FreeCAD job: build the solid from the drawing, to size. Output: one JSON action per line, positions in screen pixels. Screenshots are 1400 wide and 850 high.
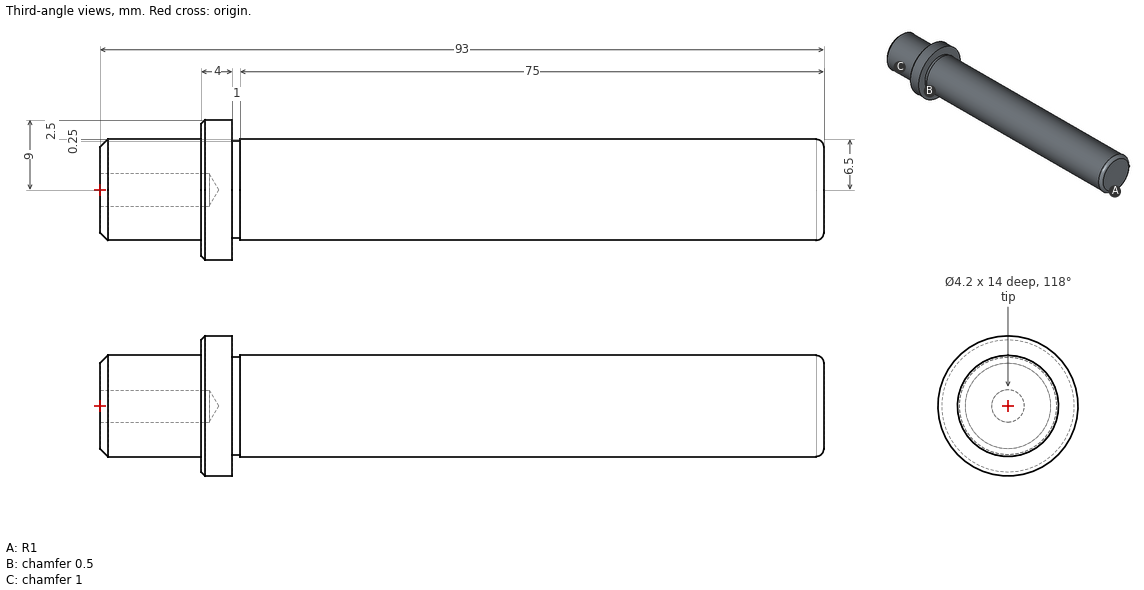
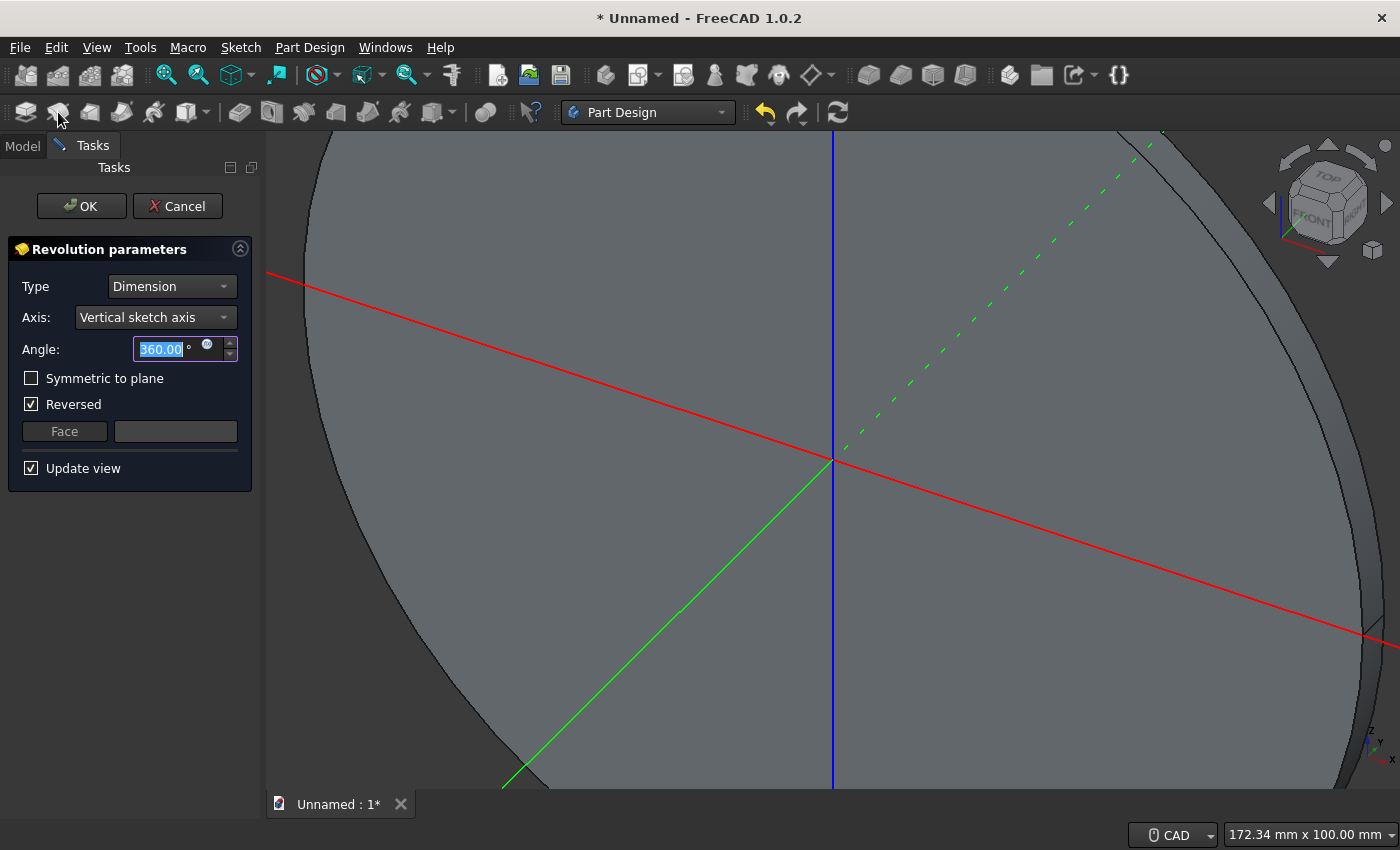
{"action": "left_click", "coordinate": [156, 318]}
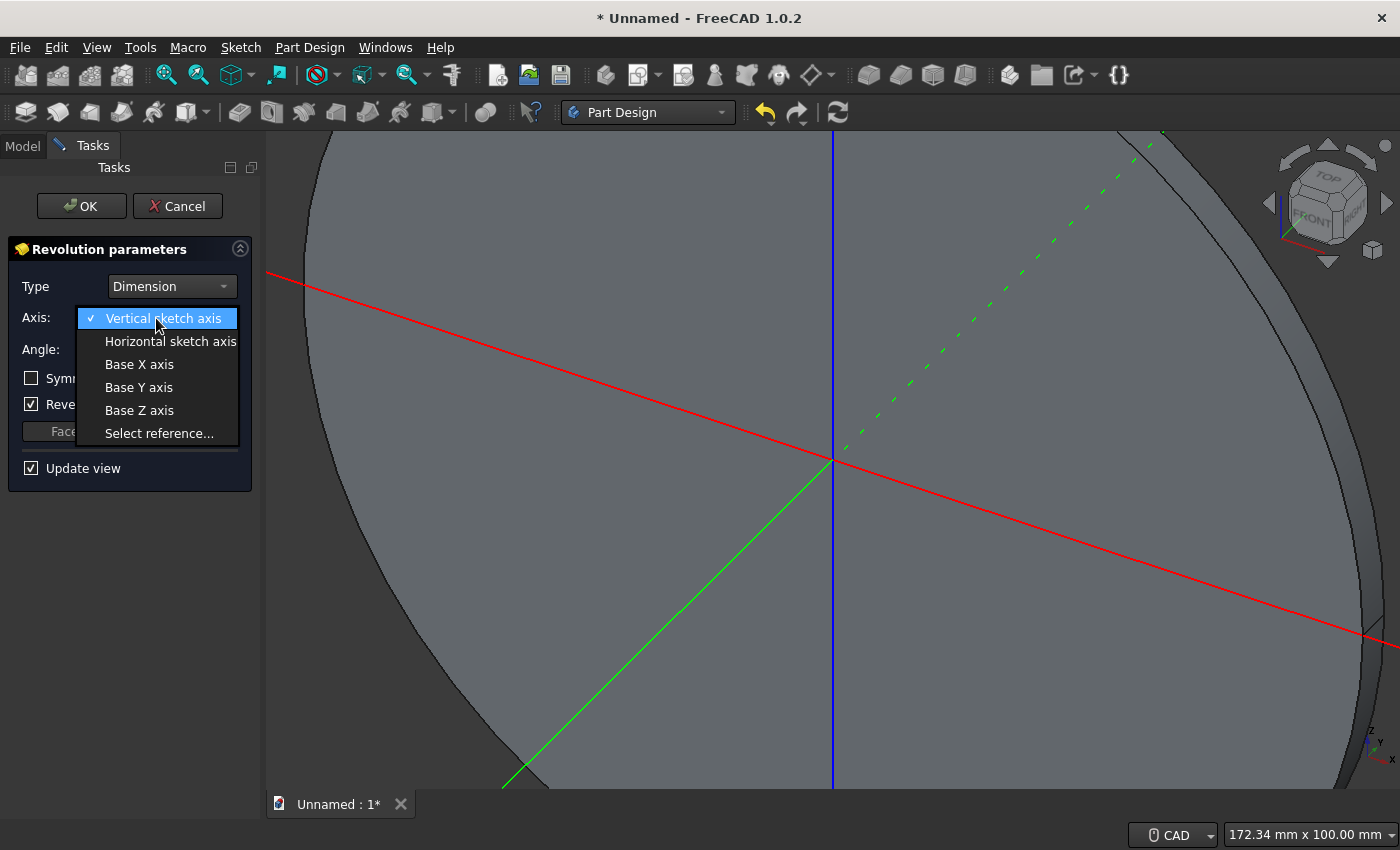
{"action": "left_click", "coordinate": [156, 342]}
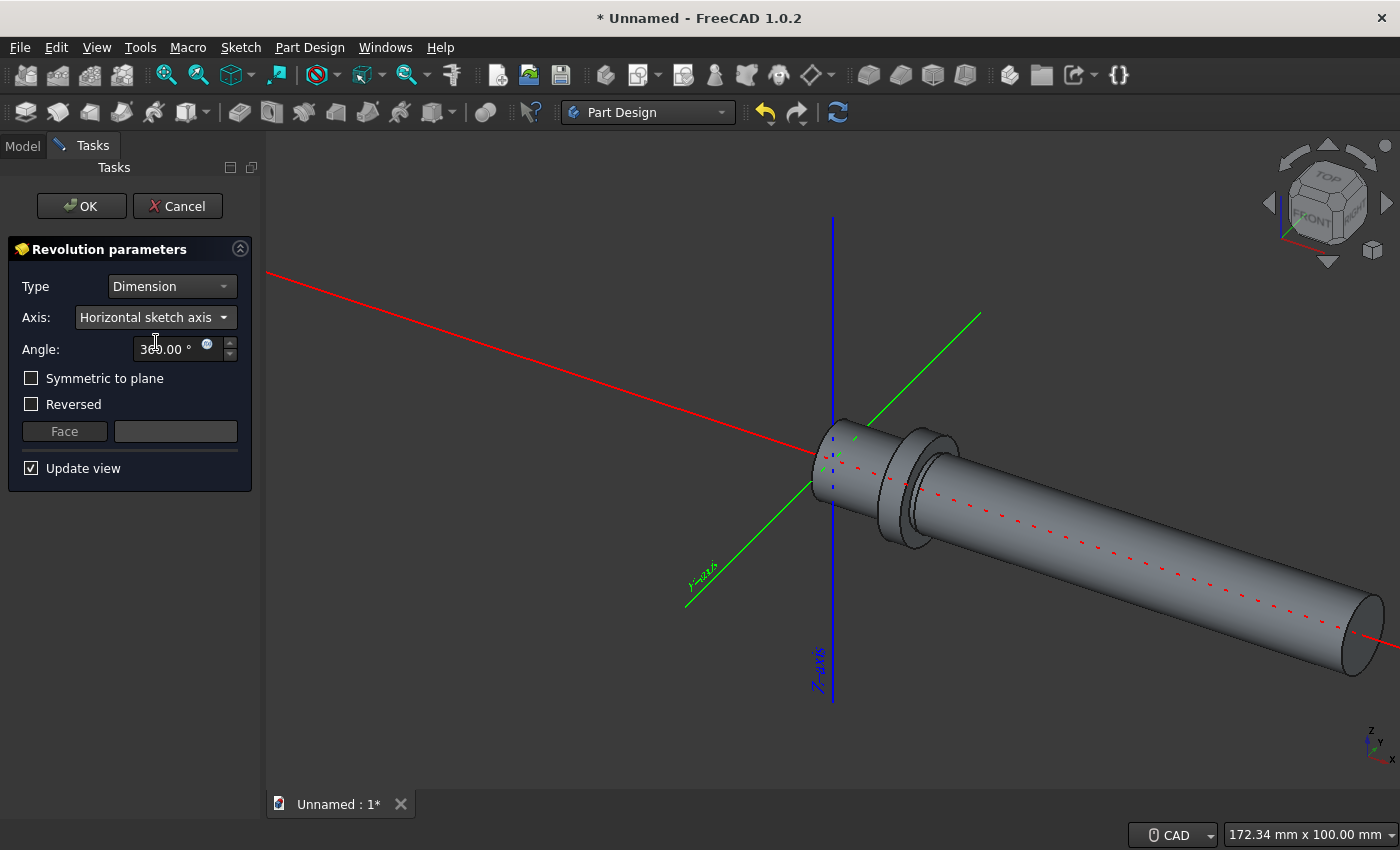
{"action": "left_click", "coordinate": [82, 206]}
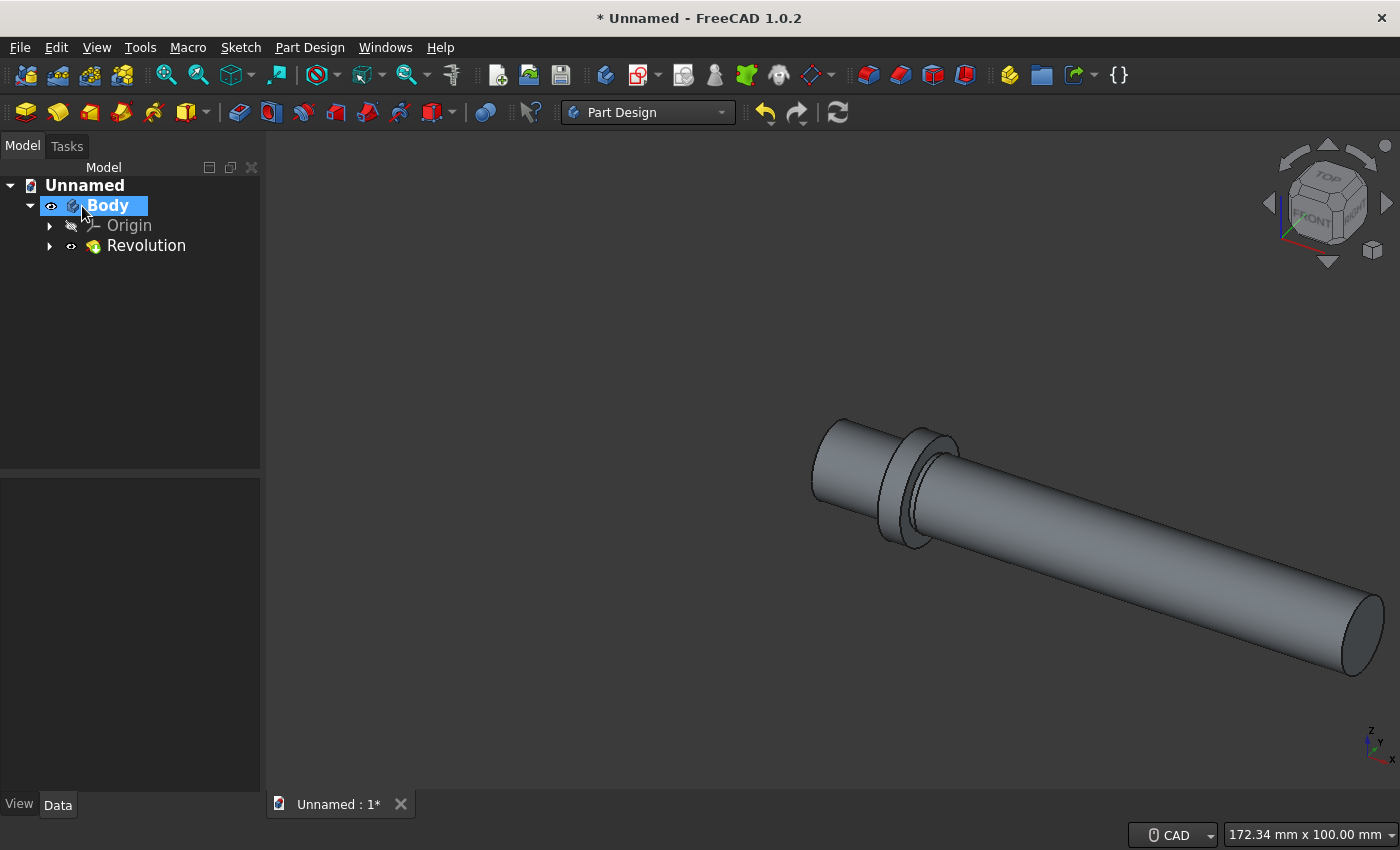
{"action": "key", "text": "0"}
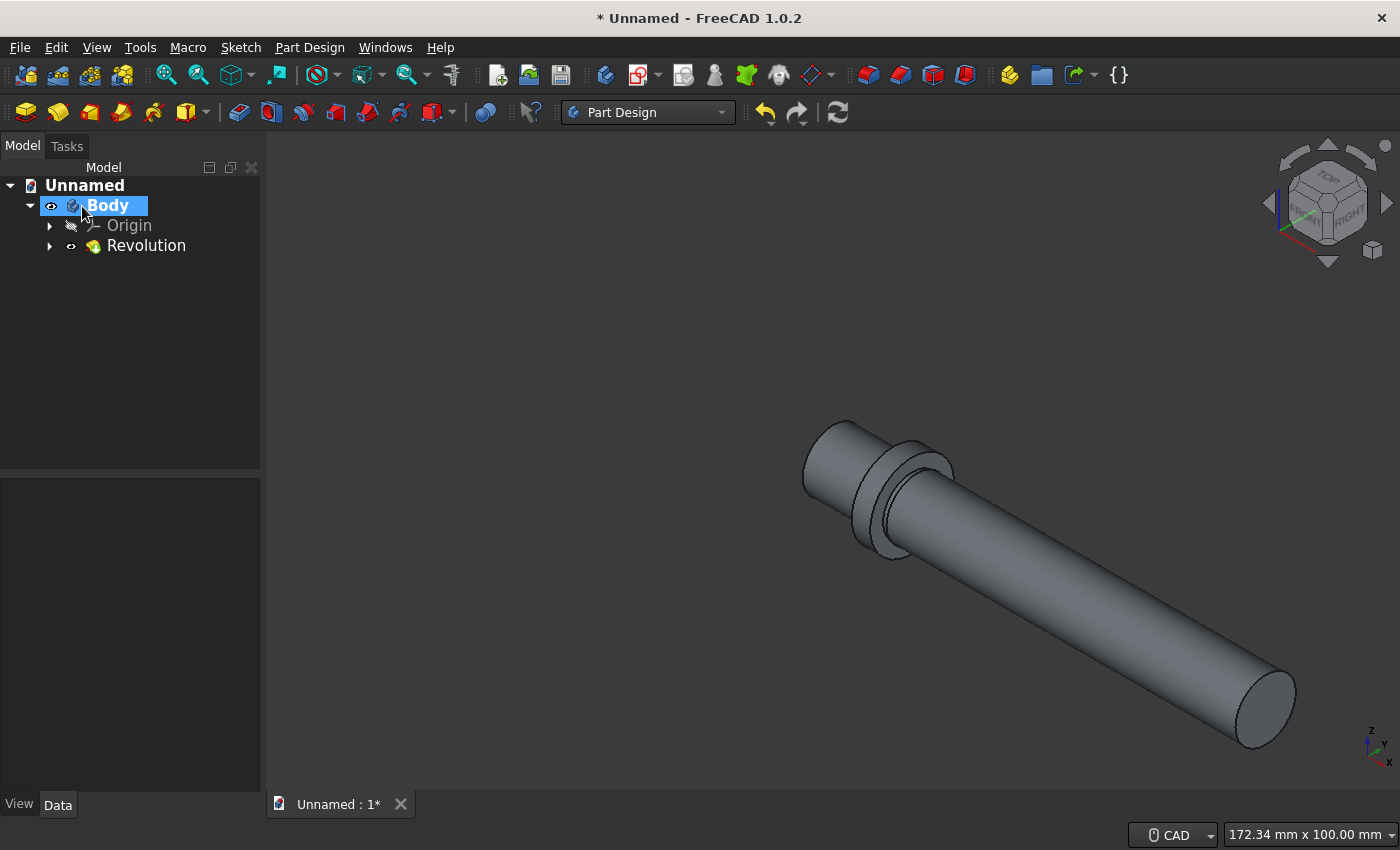
{"action": "left_click", "coordinate": [1235, 726]}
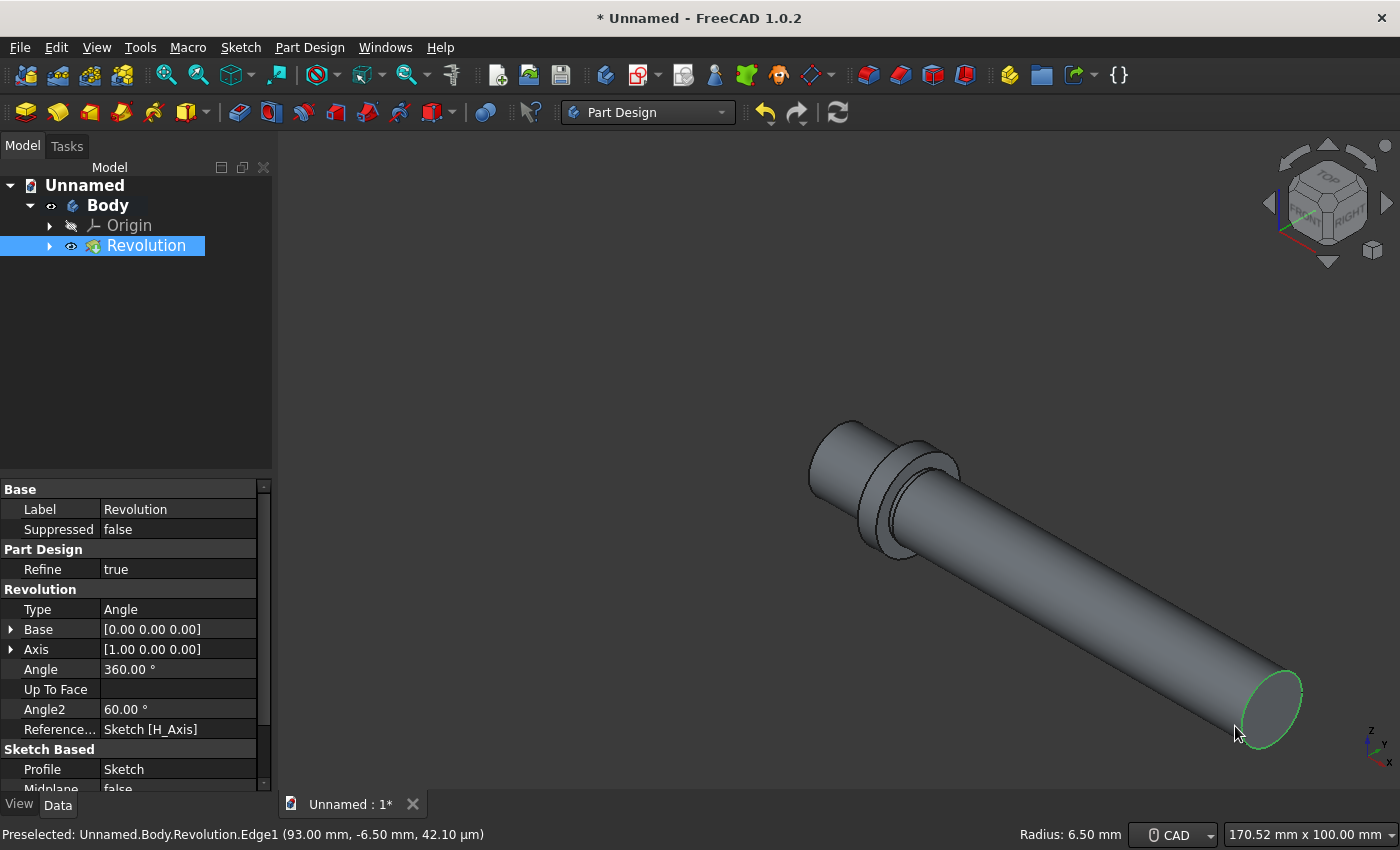
{"action": "left_click", "coordinate": [870, 76]}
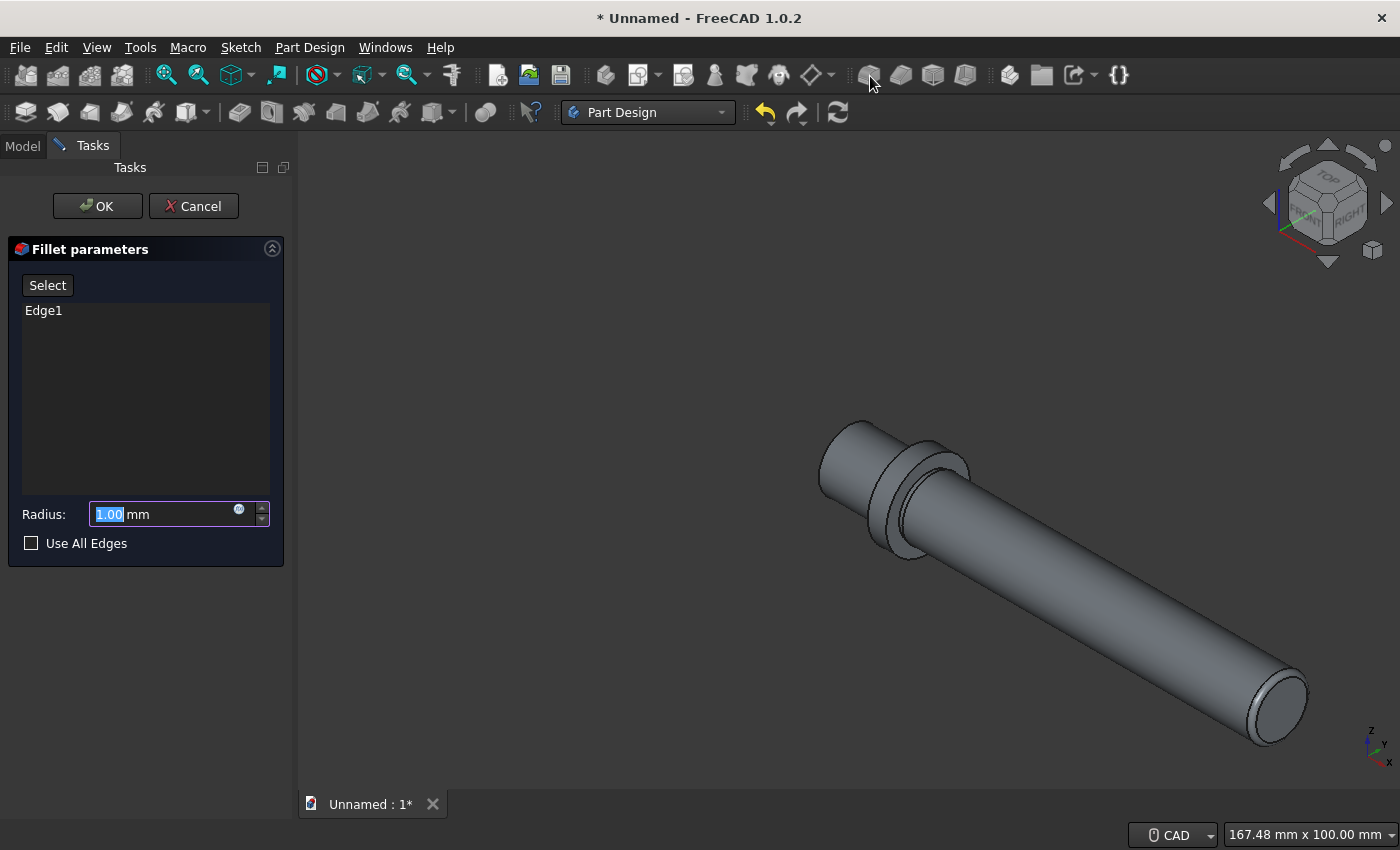
{"action": "type", "text": "1"}
{"action": "key", "text": "Tab"}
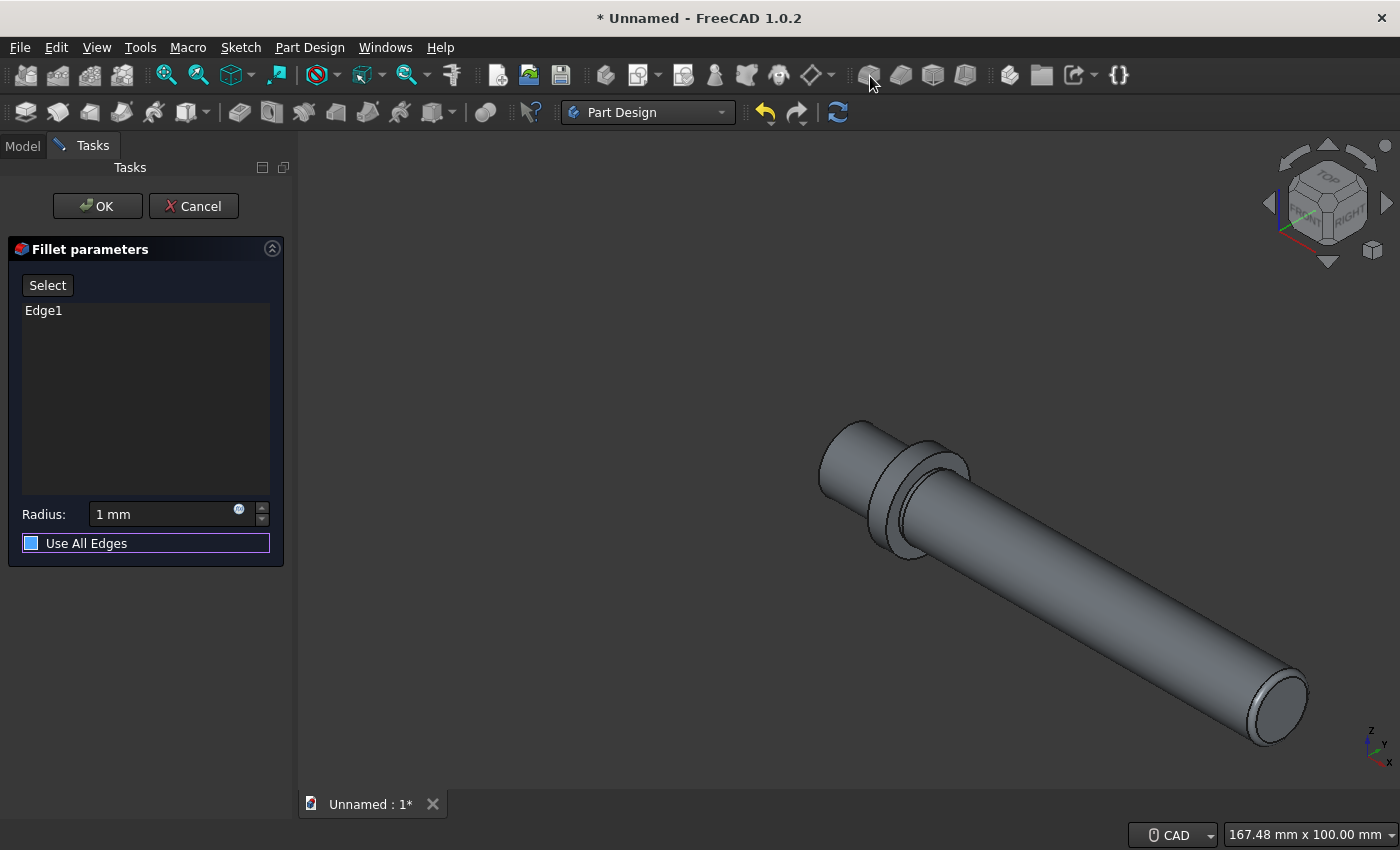
{"action": "left_click", "coordinate": [98, 206]}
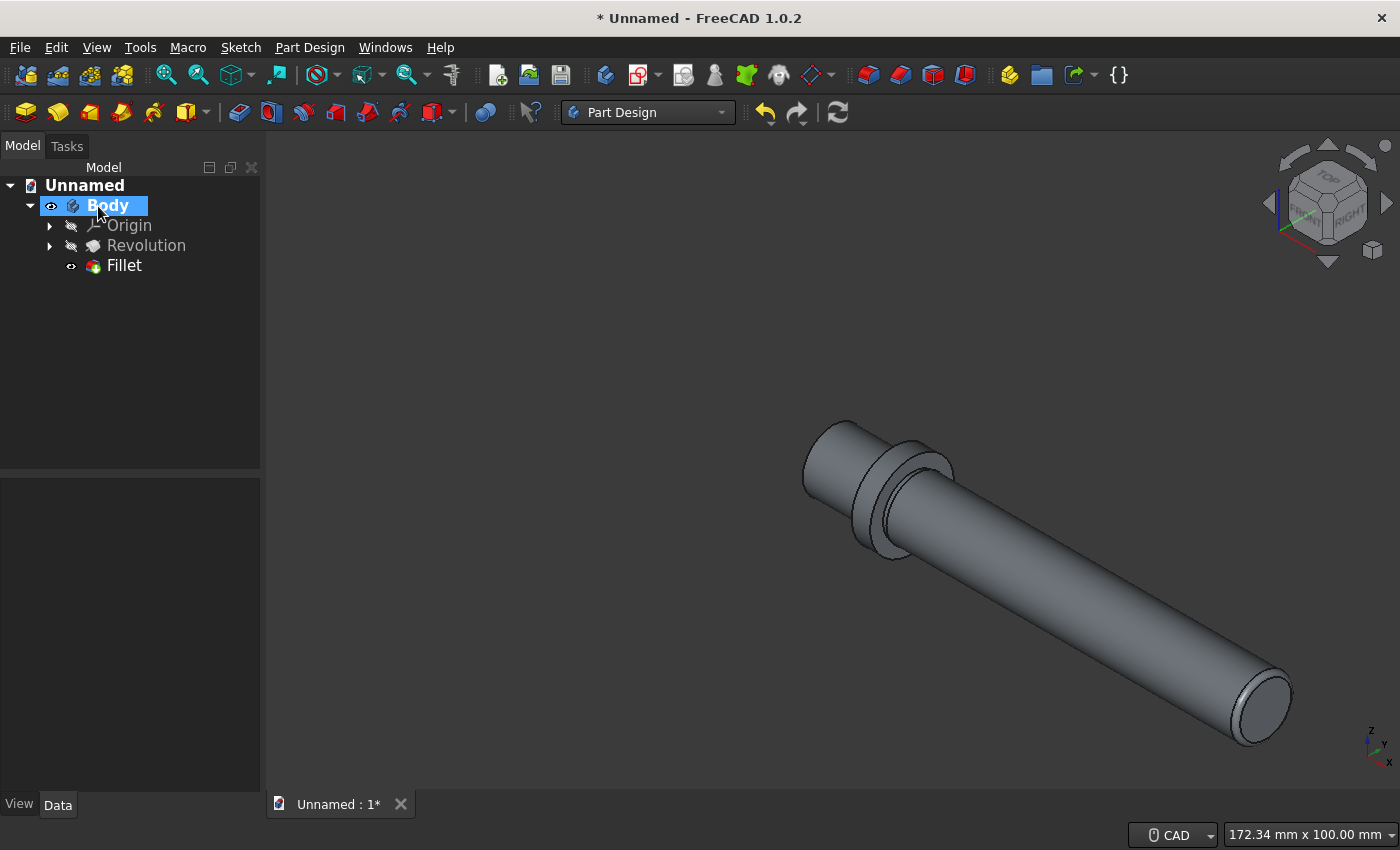
{"action": "left_click", "coordinate": [906, 440]}